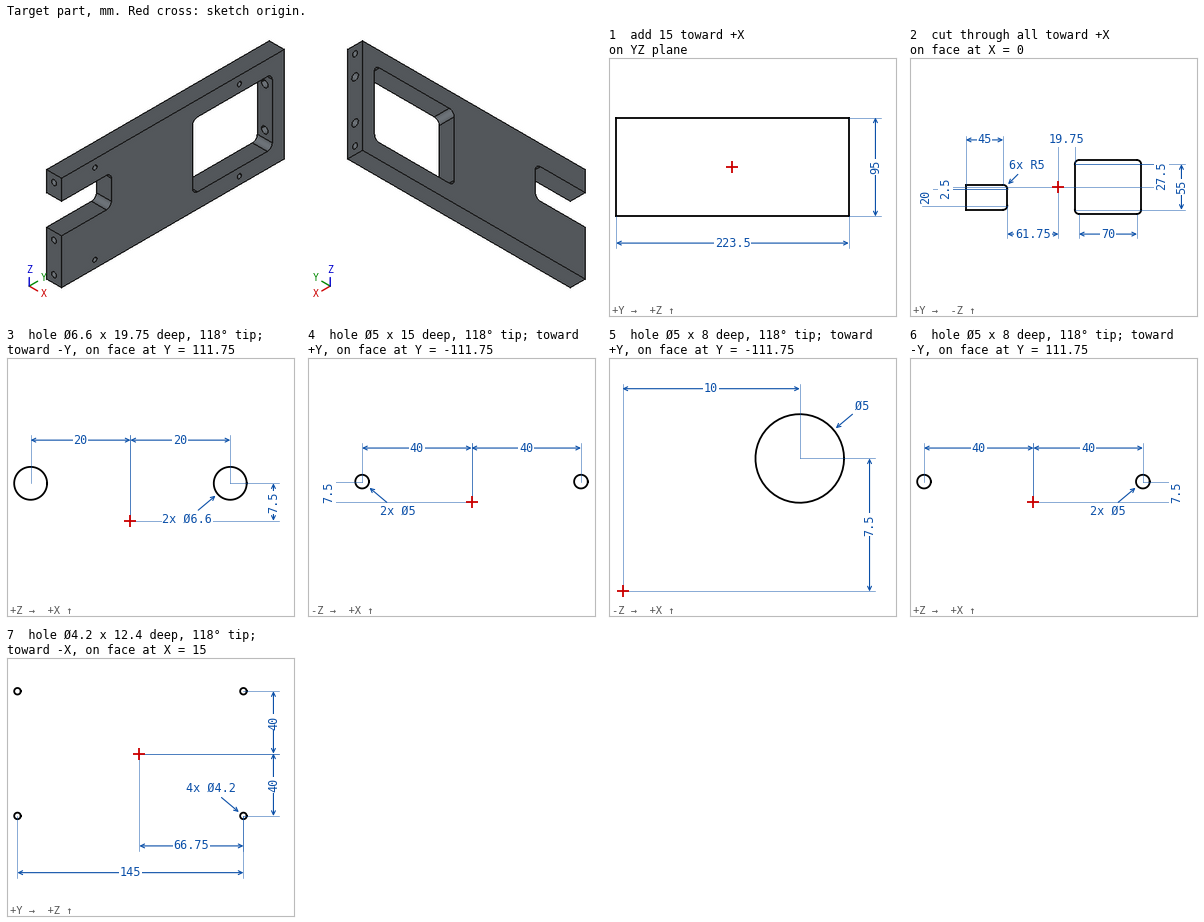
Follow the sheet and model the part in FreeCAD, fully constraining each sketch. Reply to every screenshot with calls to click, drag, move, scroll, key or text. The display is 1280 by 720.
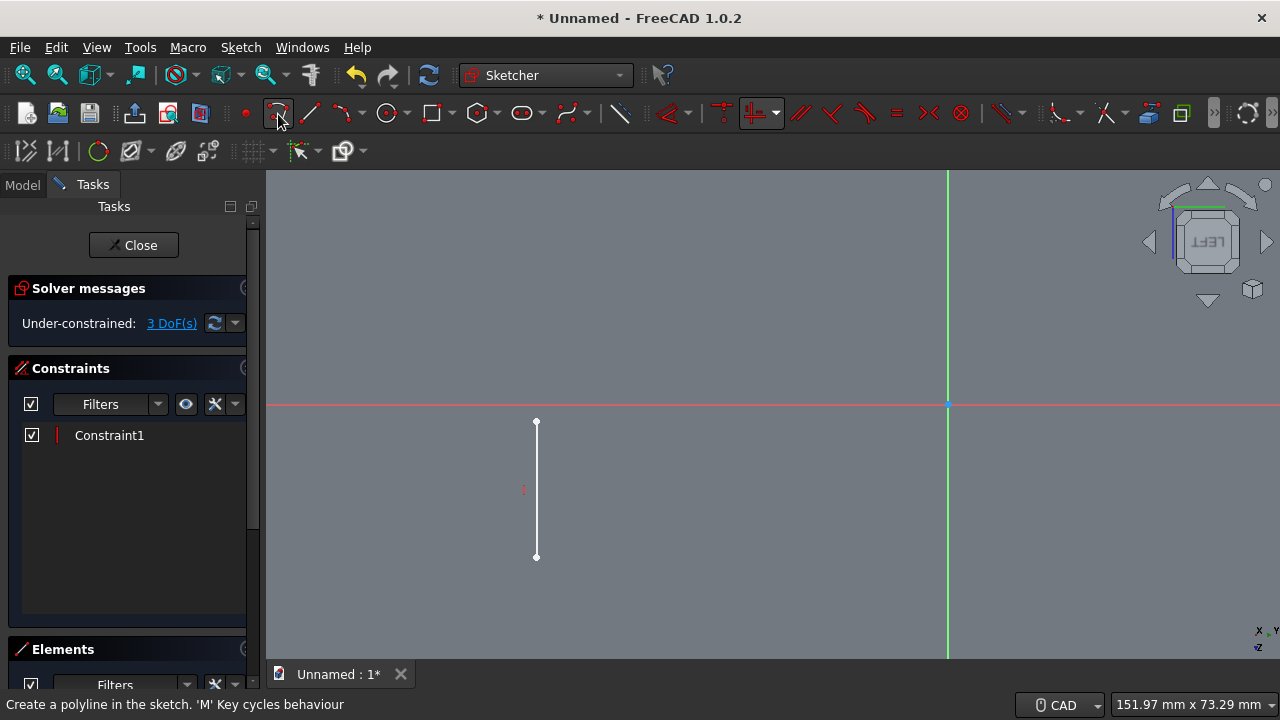
click(503, 388)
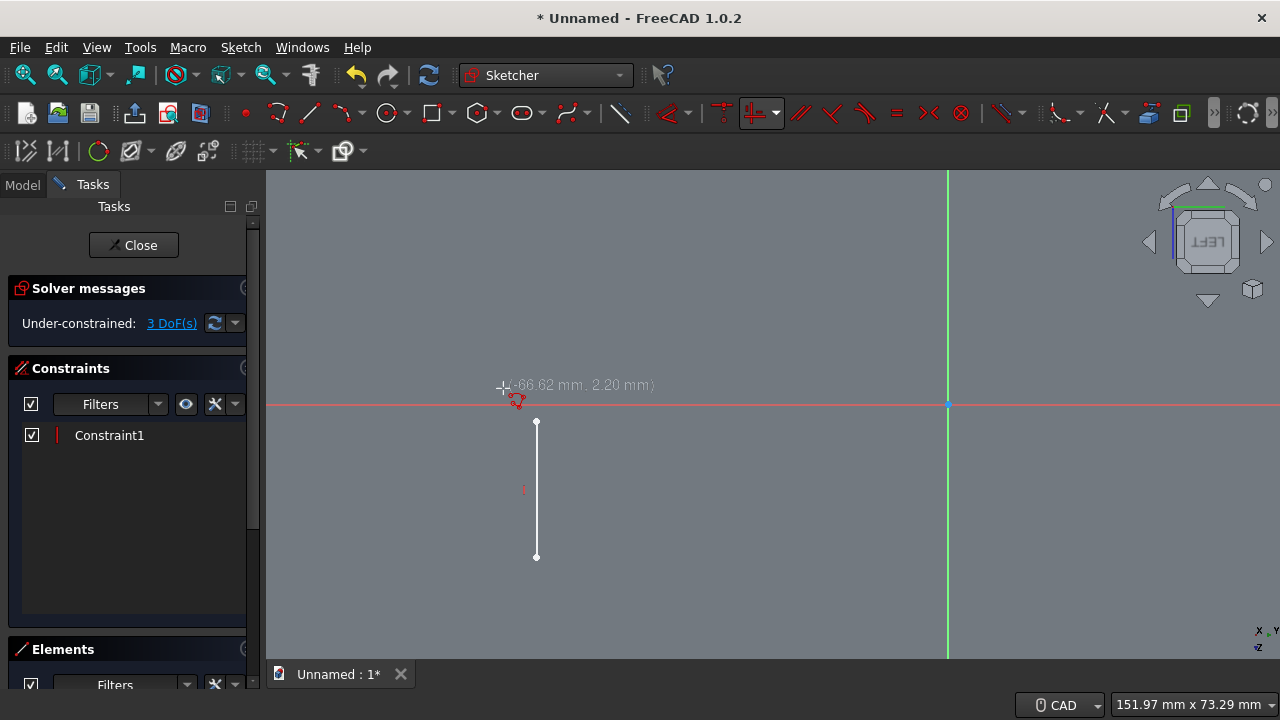
scroll(538, 423, down, 4)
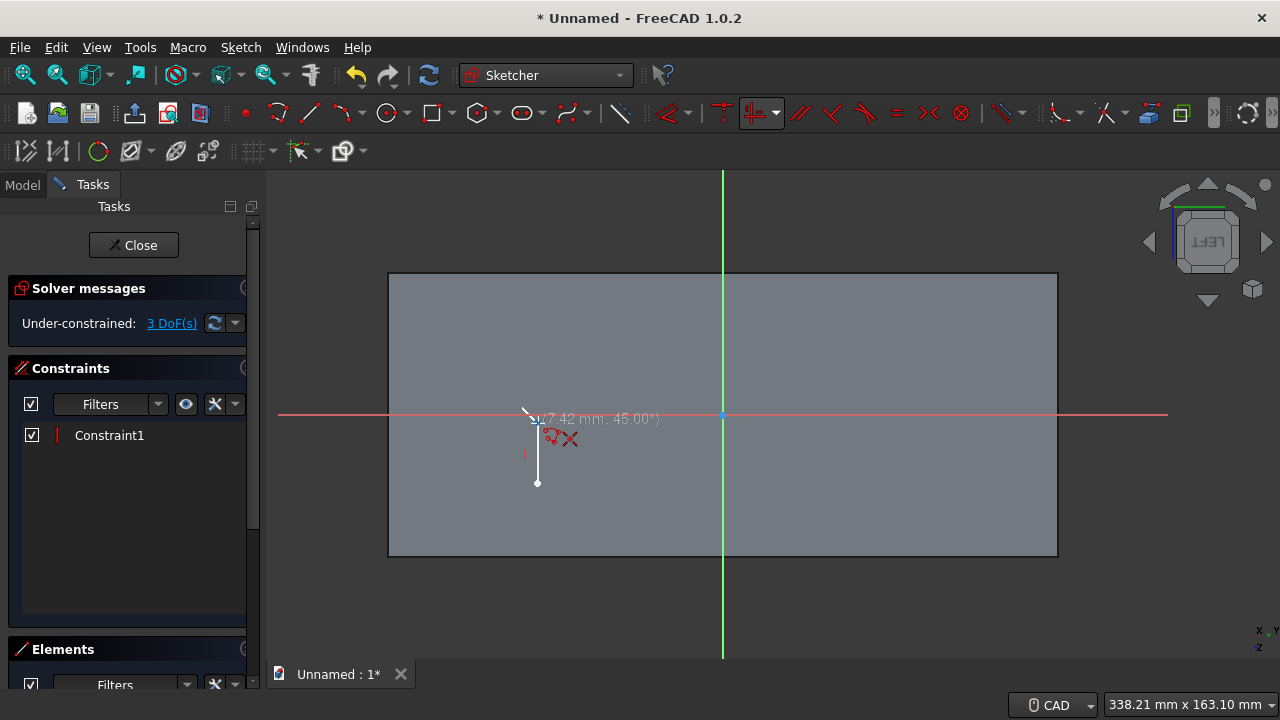
scroll(388, 408, up, 4)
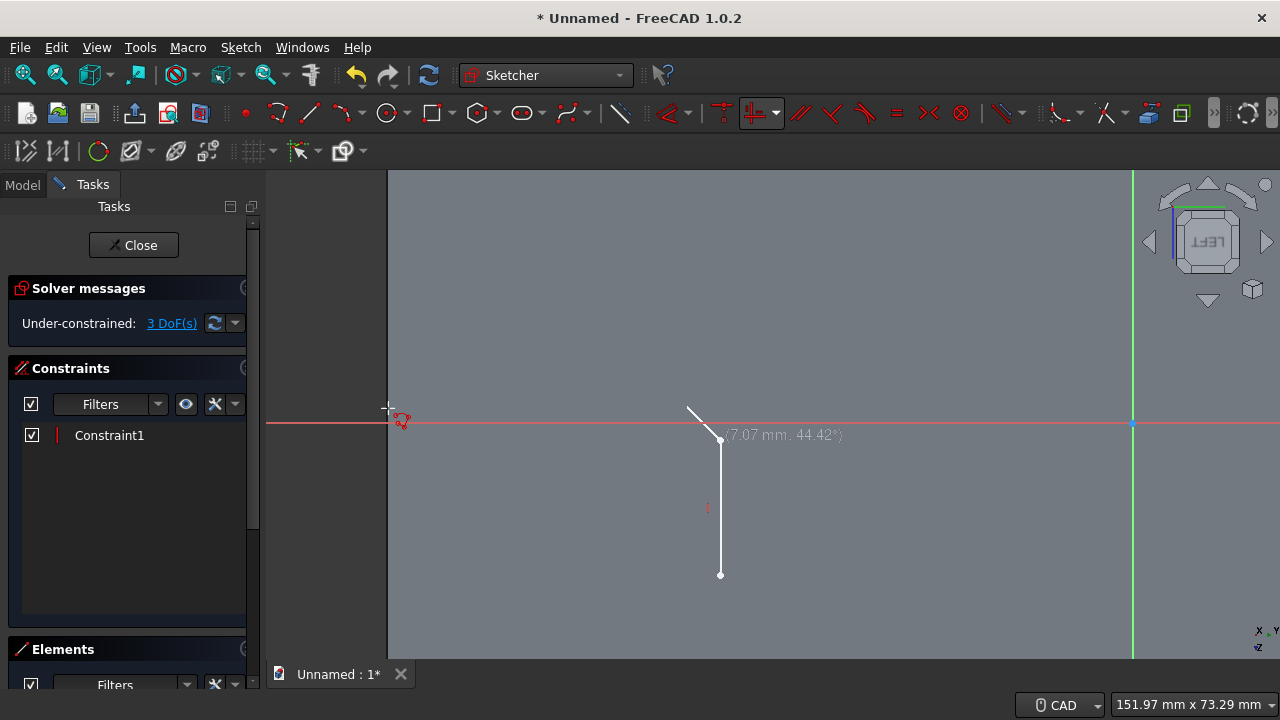
click(387, 406)
click(387, 607)
click(687, 607)
right_click(687, 607)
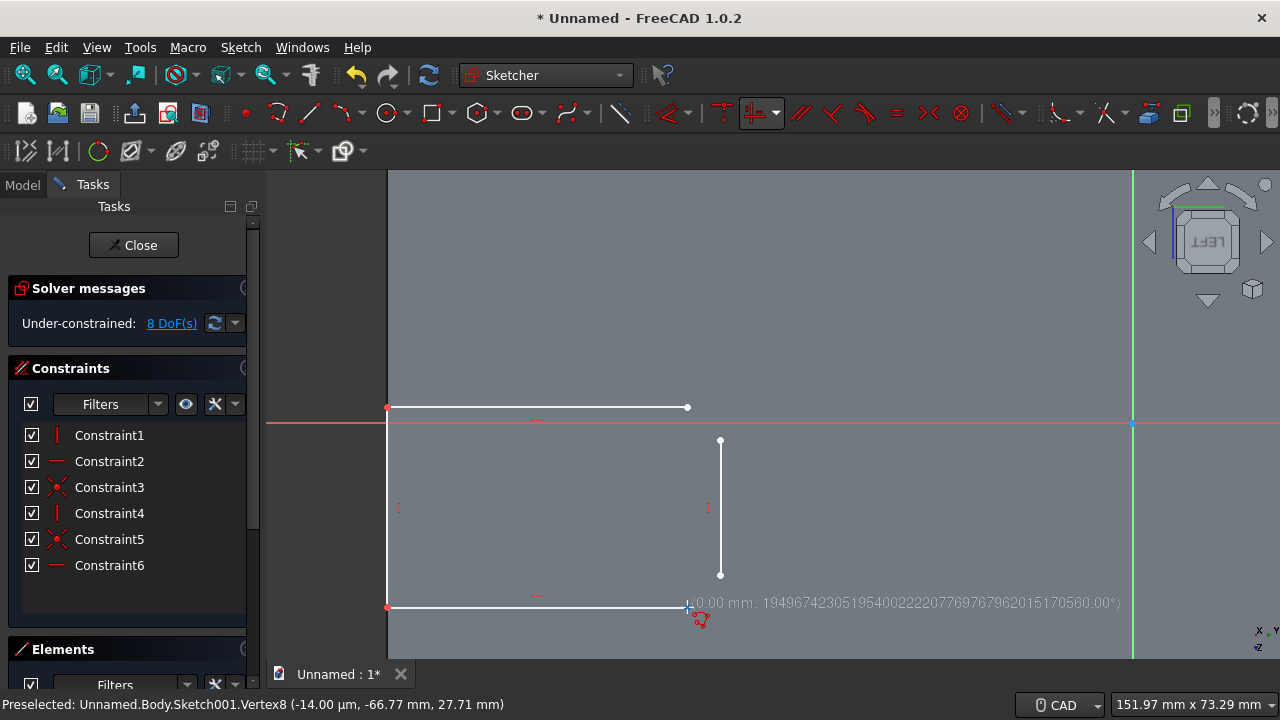
click(342, 114)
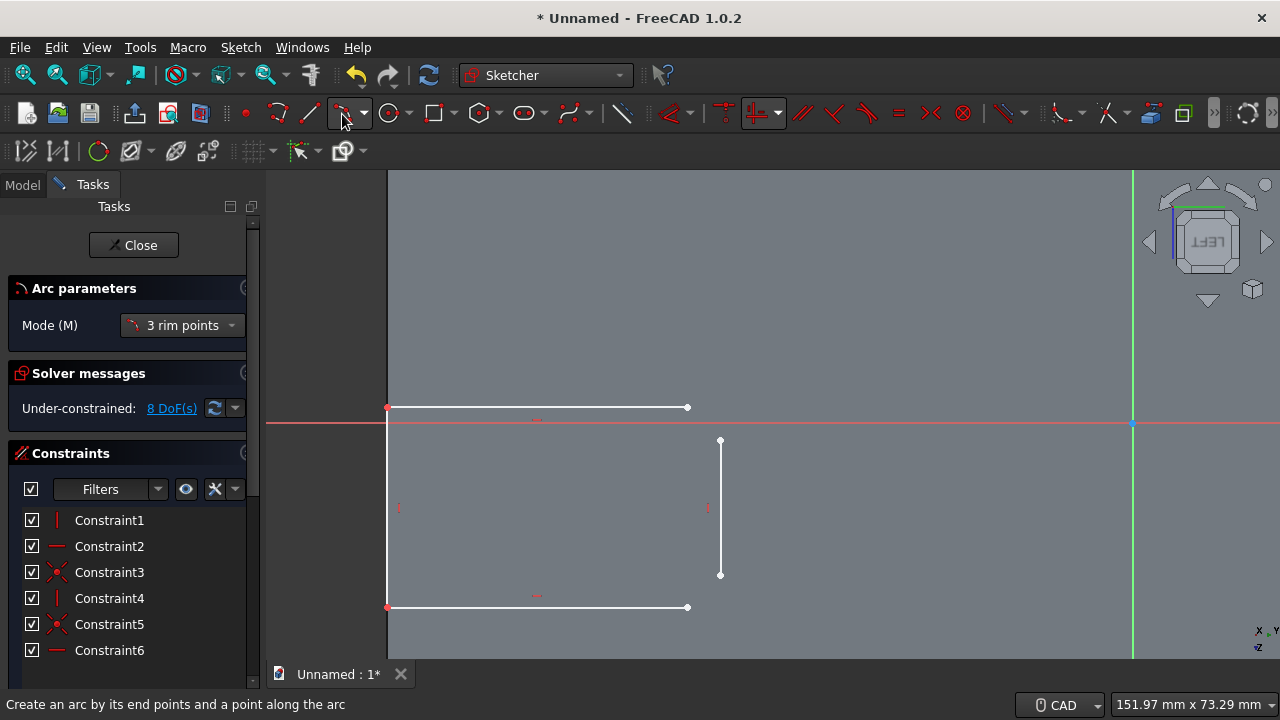
click(721, 440)
click(687, 407)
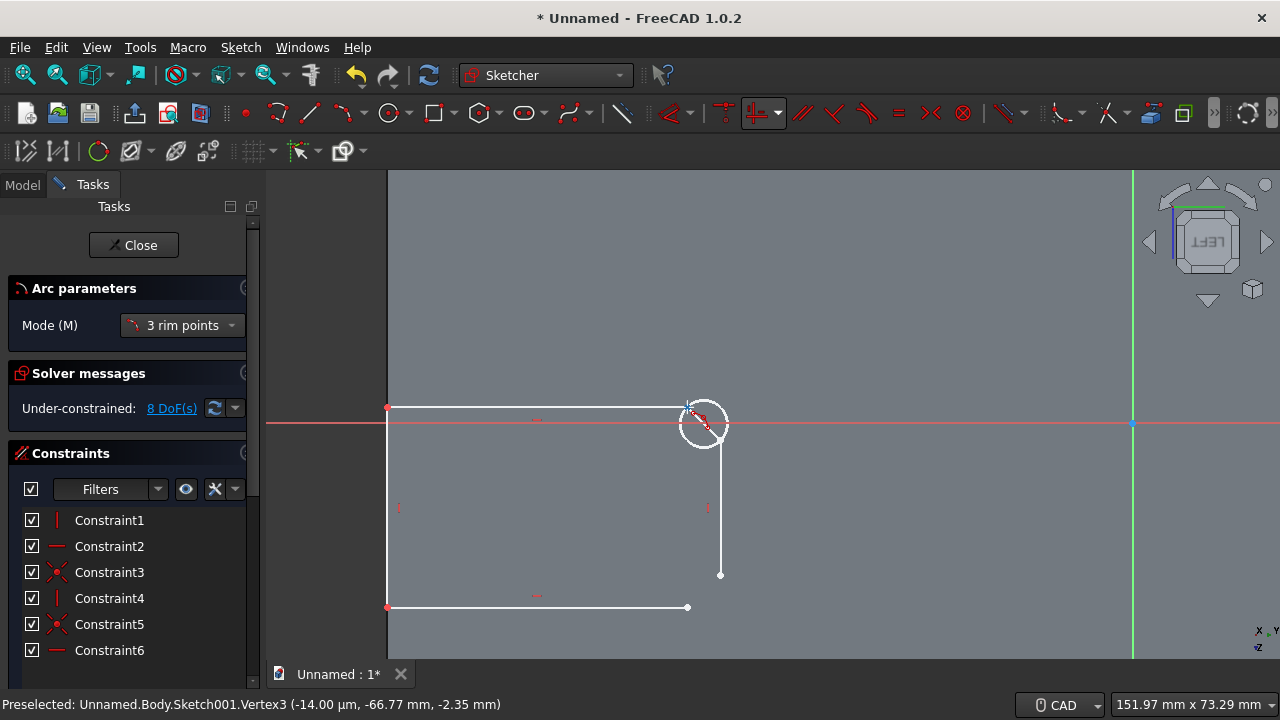
scroll(707, 413, up, 3)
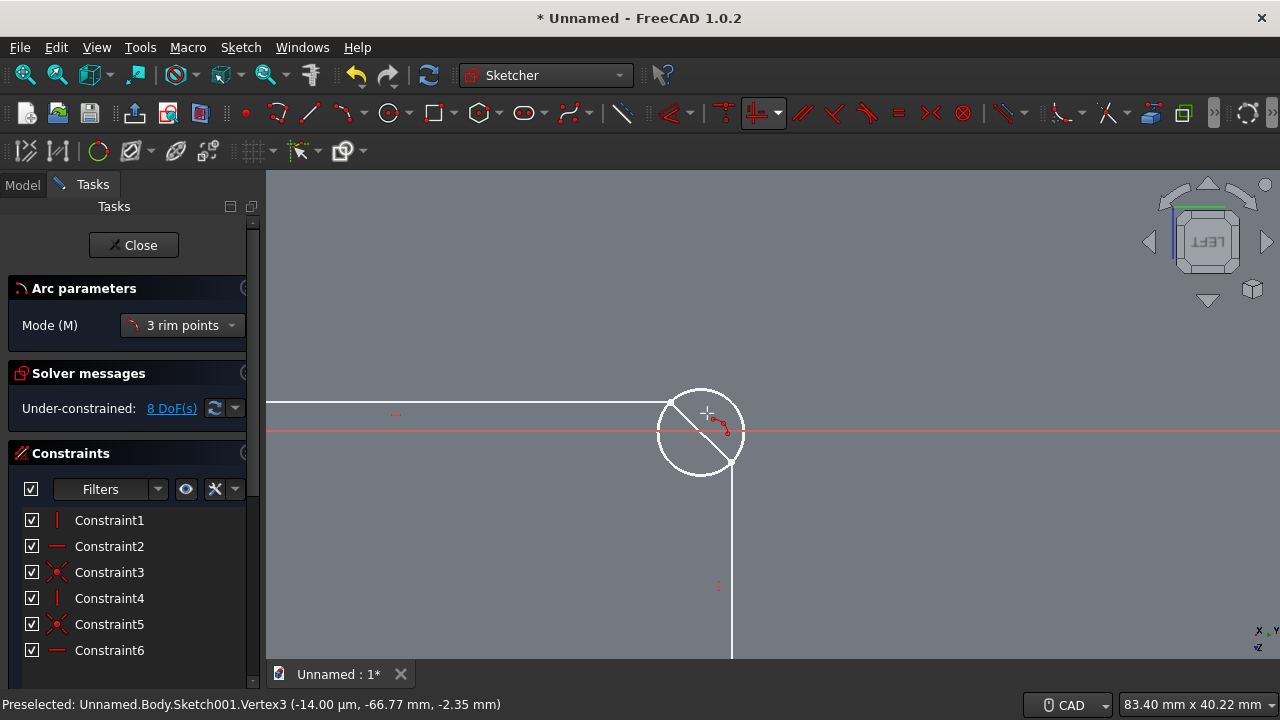
click(706, 412)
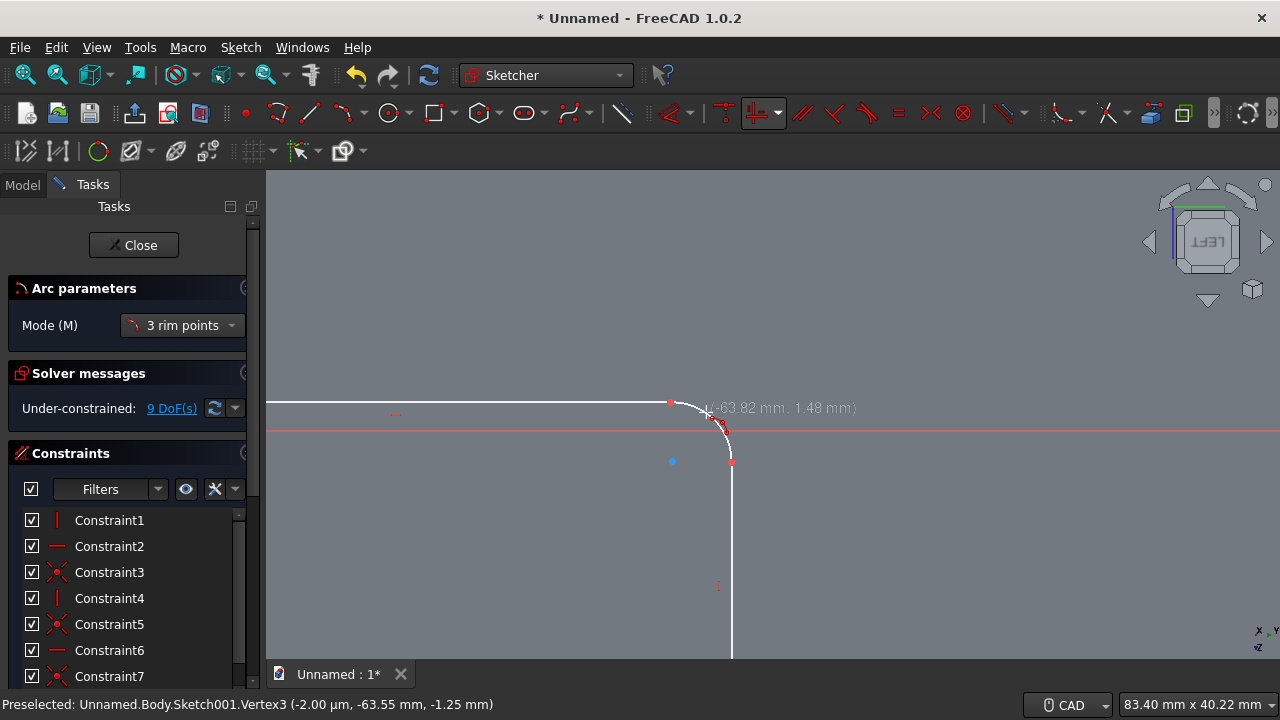
scroll(474, 409, down, 7)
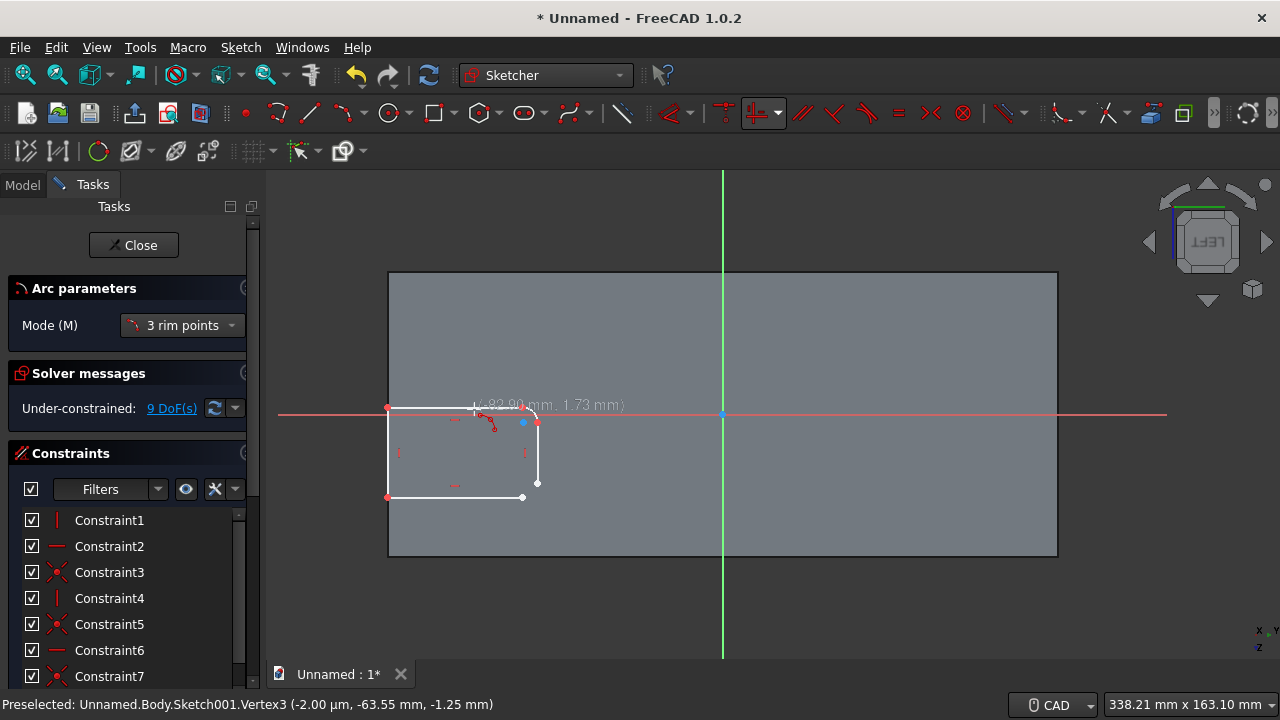
click(523, 498)
click(538, 483)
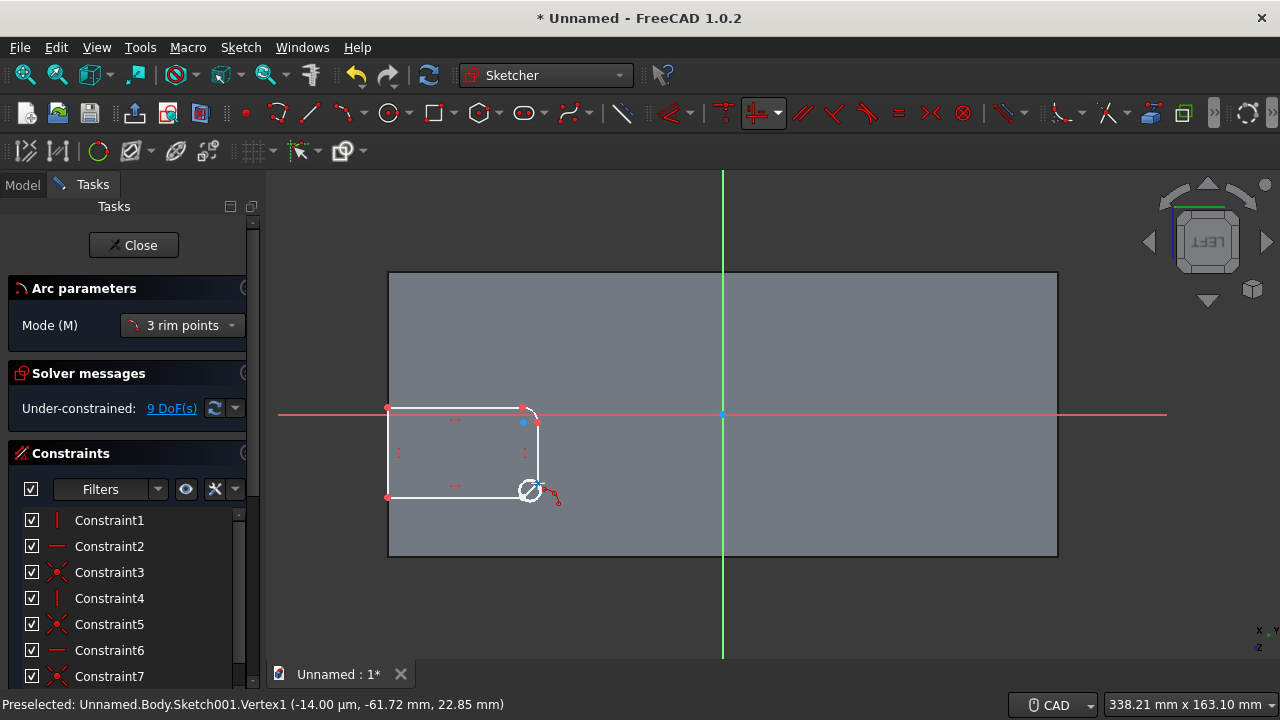
scroll(533, 493, up, 7)